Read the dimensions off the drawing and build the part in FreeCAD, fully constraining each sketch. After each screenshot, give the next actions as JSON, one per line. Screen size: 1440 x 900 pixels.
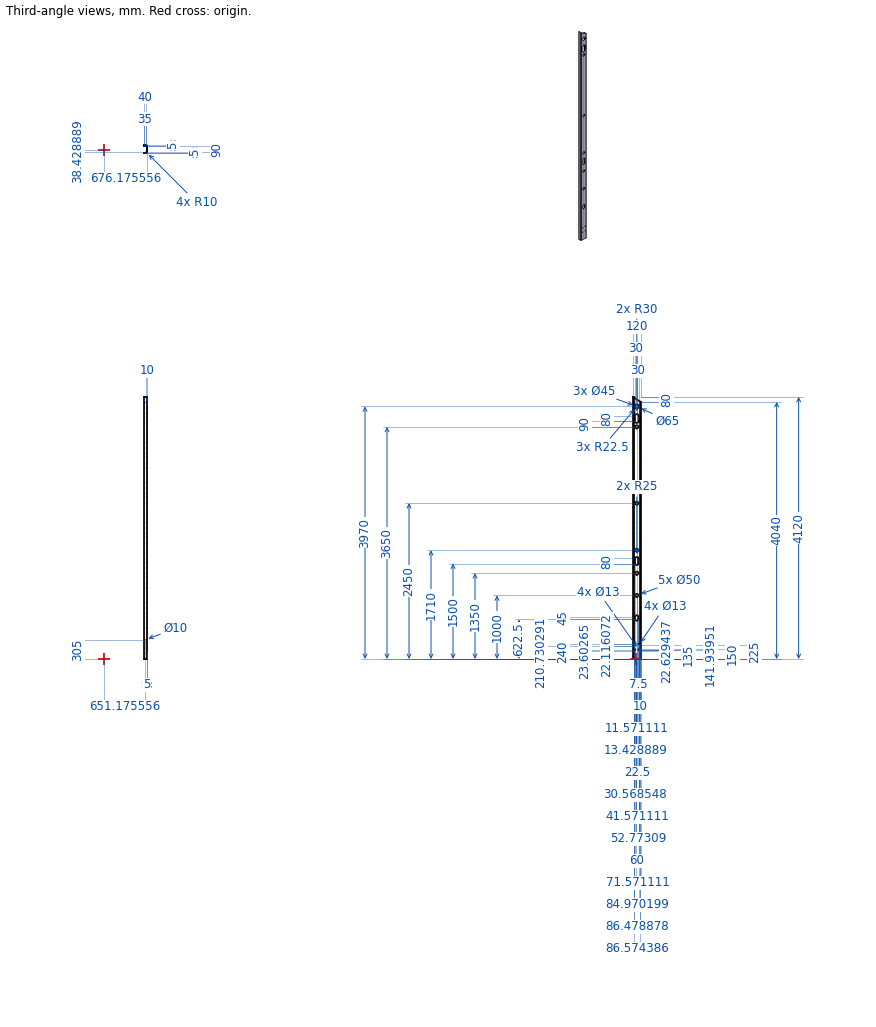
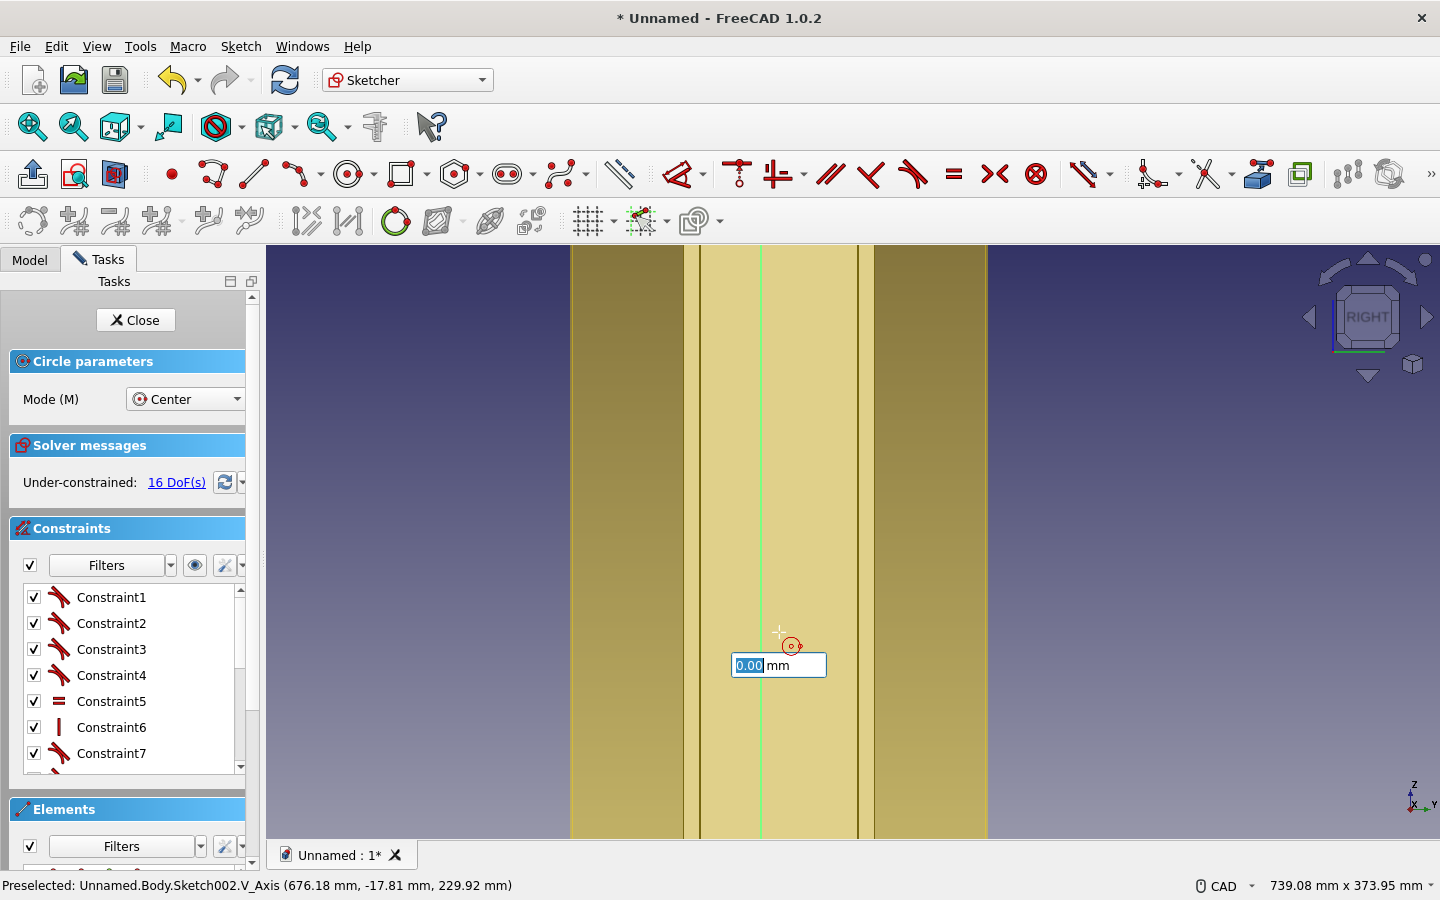
{"action": "scroll", "coordinate": [785, 639], "scroll_direction": "down", "scroll_amount": 14}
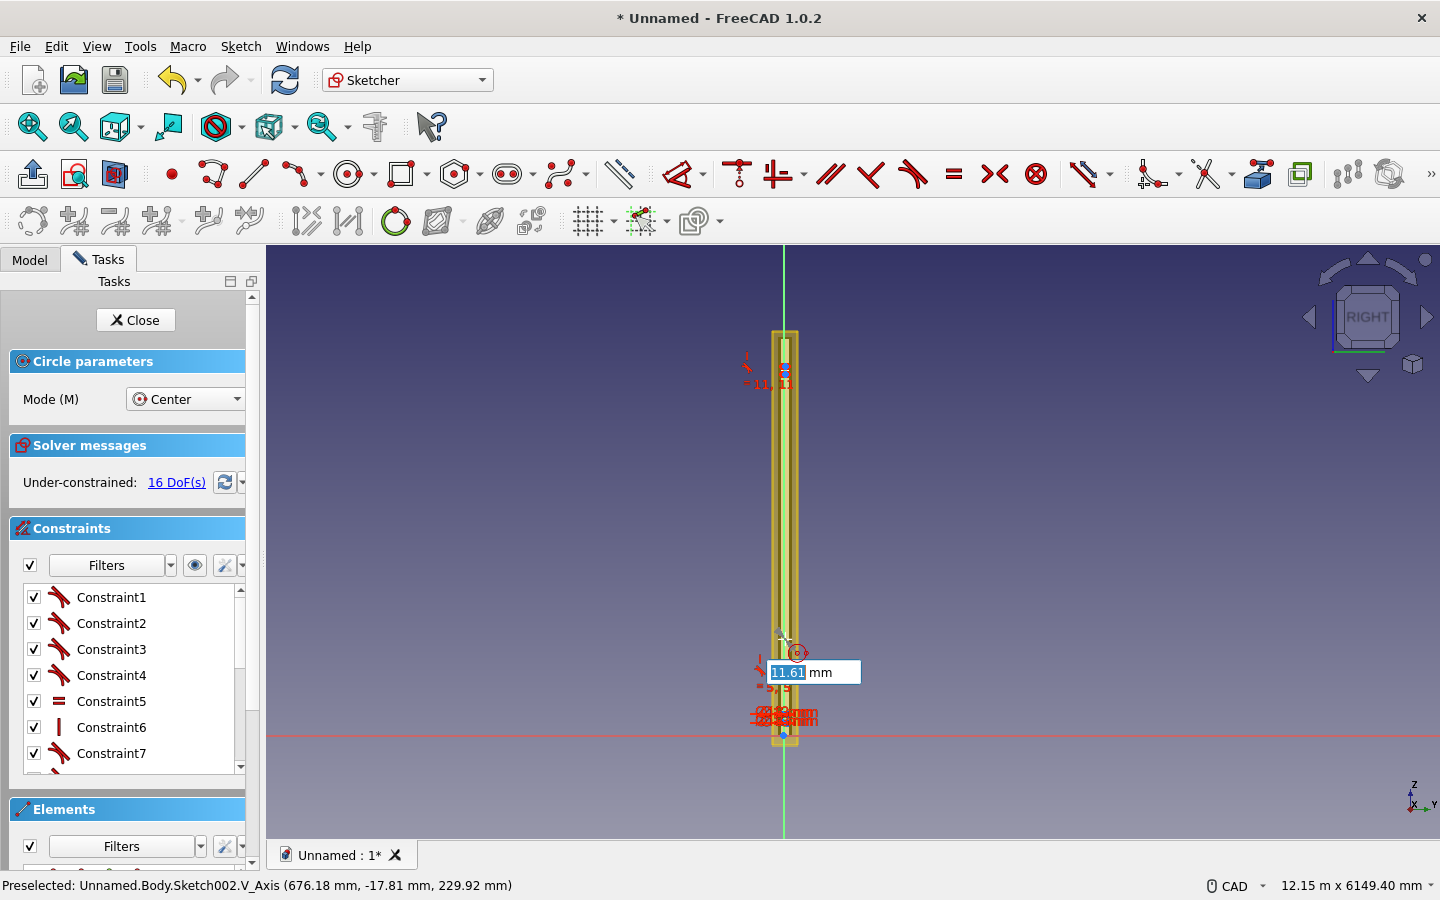
{"action": "scroll", "coordinate": [787, 638], "scroll_direction": "up", "scroll_amount": 9}
{"action": "mouse_move", "coordinate": [783, 632]}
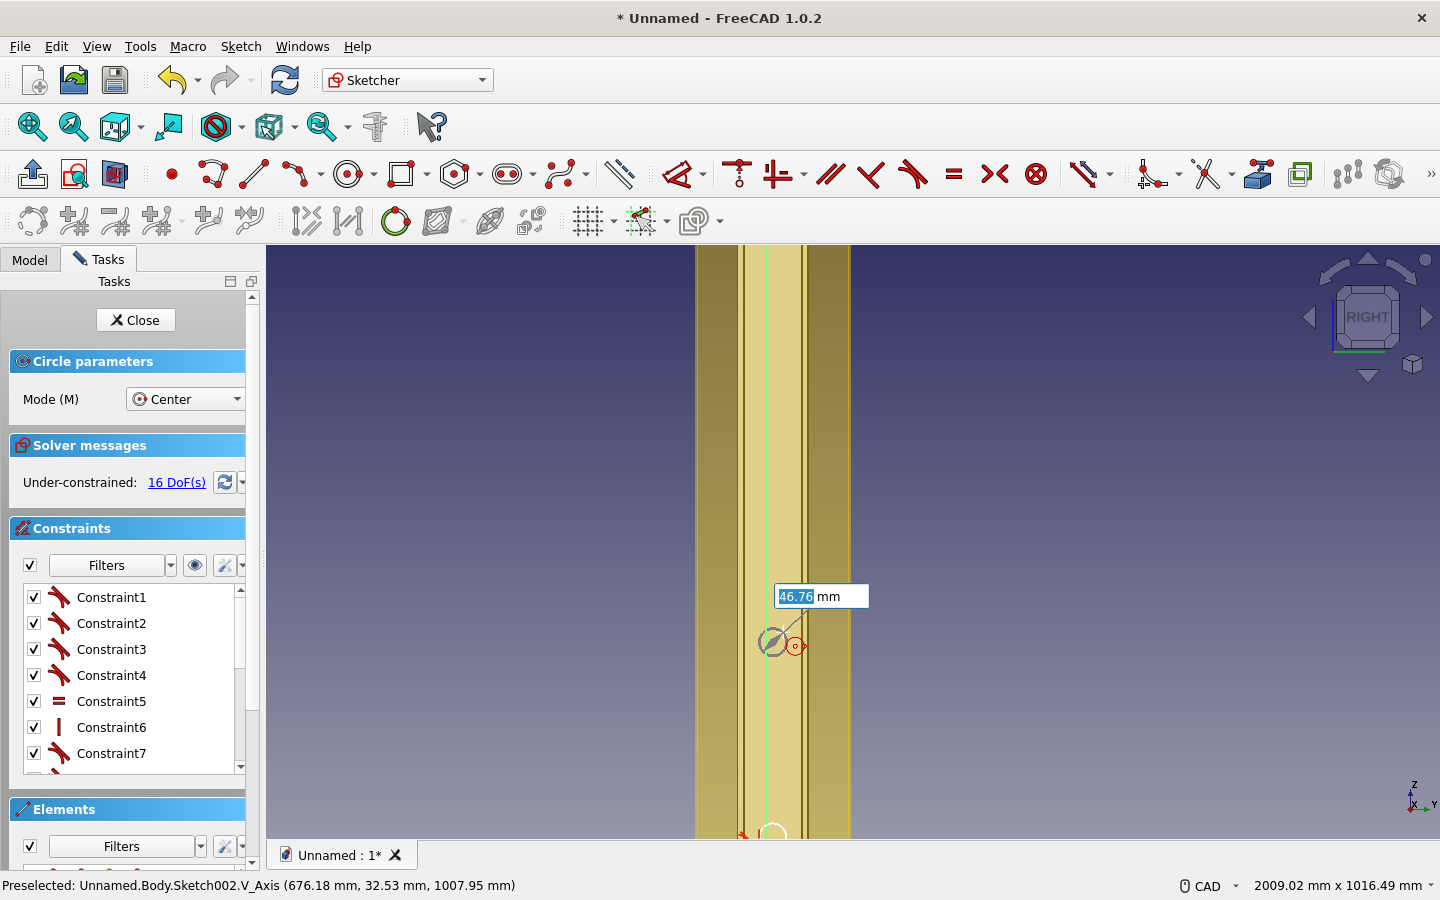
{"action": "type", "text": "50"}
{"action": "key", "text": "Return"}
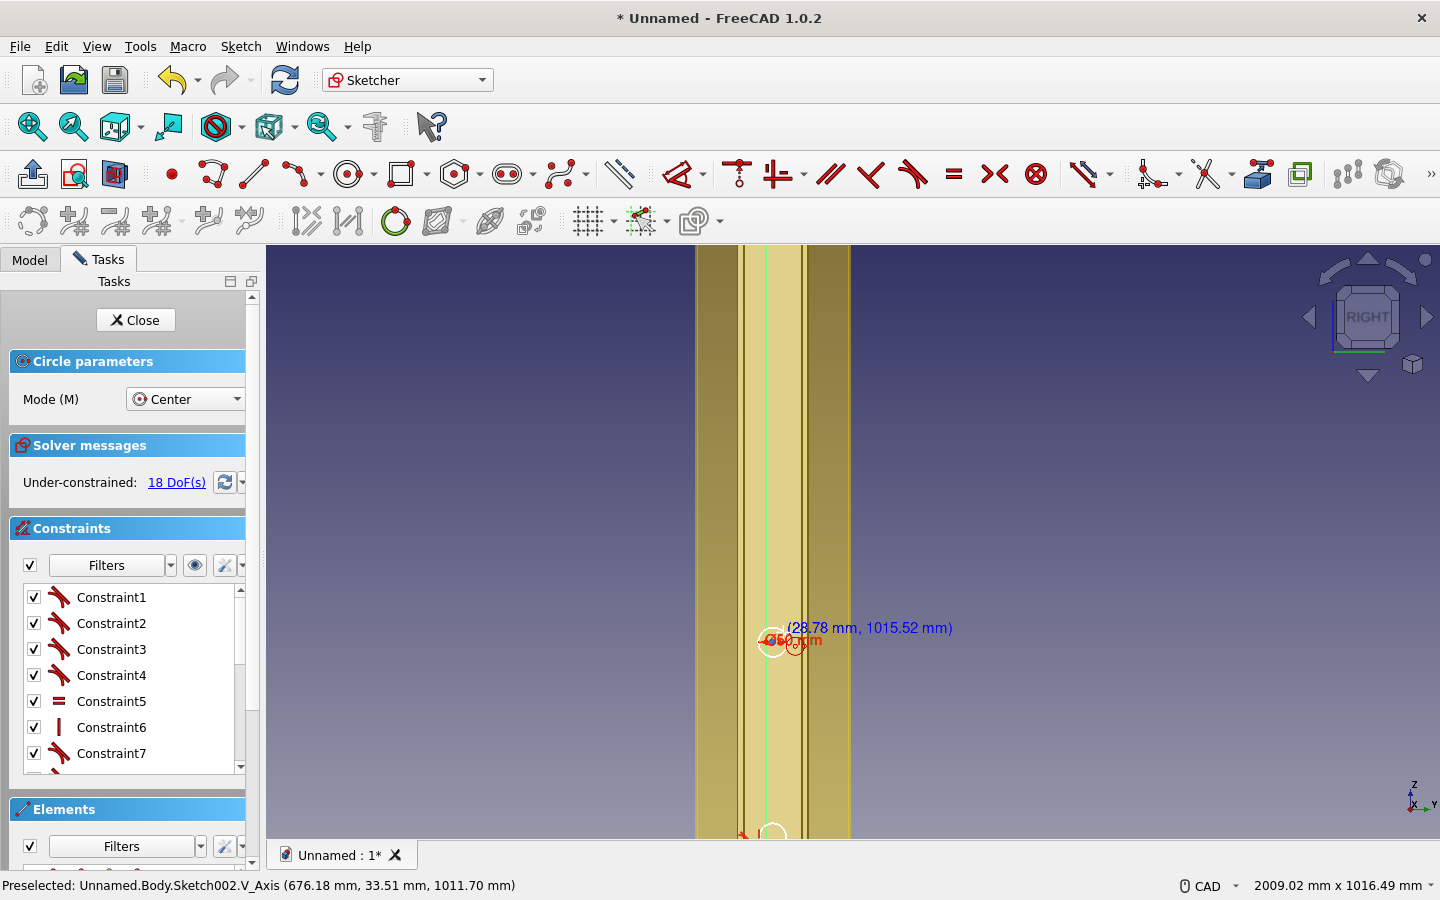
{"action": "scroll", "coordinate": [773, 438], "scroll_direction": "up", "scroll_amount": 5}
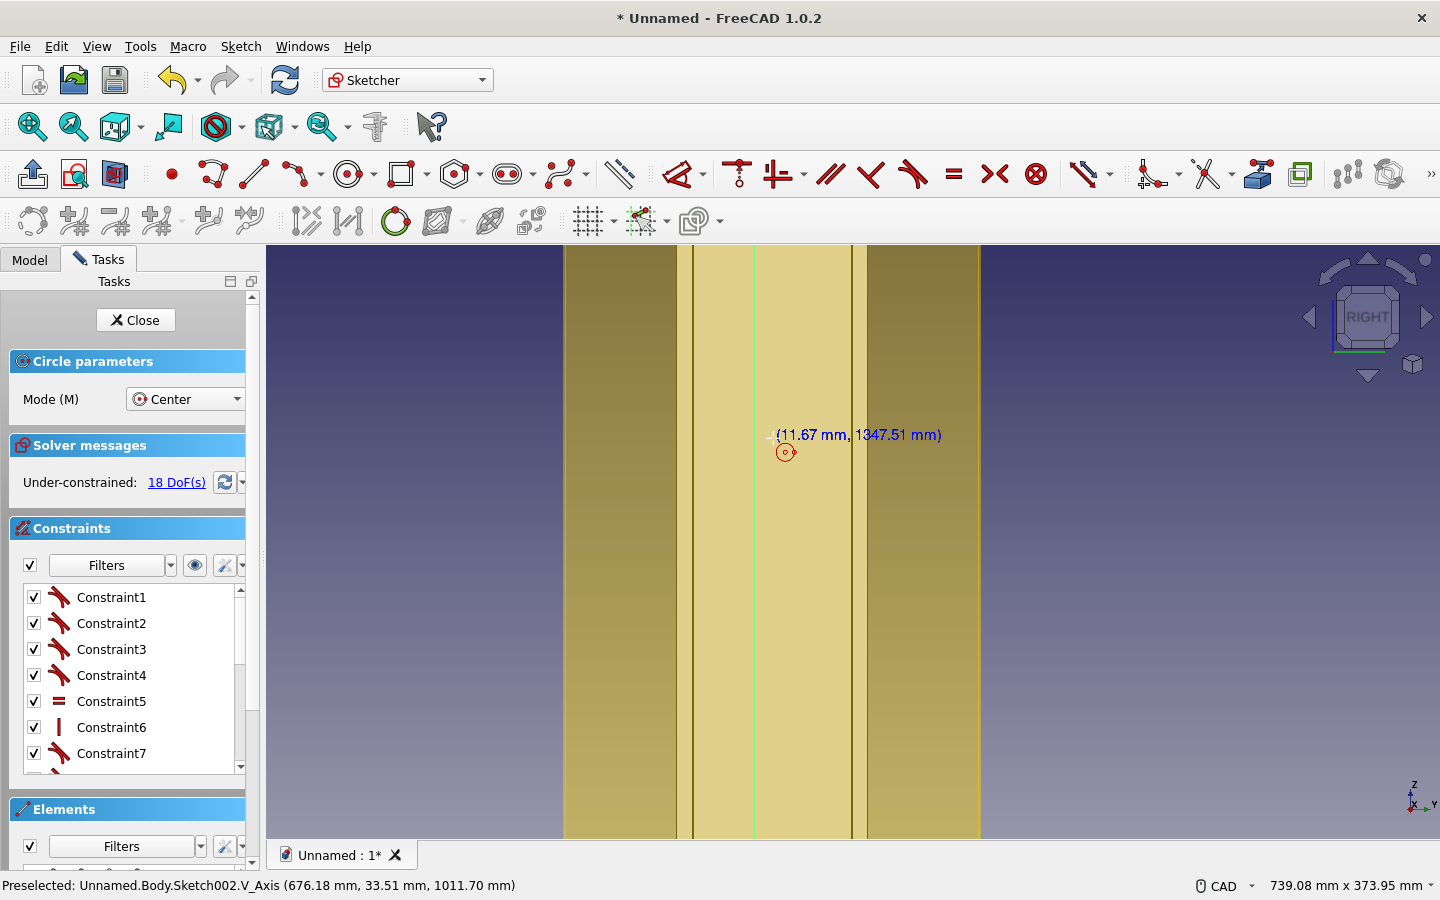
{"action": "left_click", "coordinate": [772, 436]}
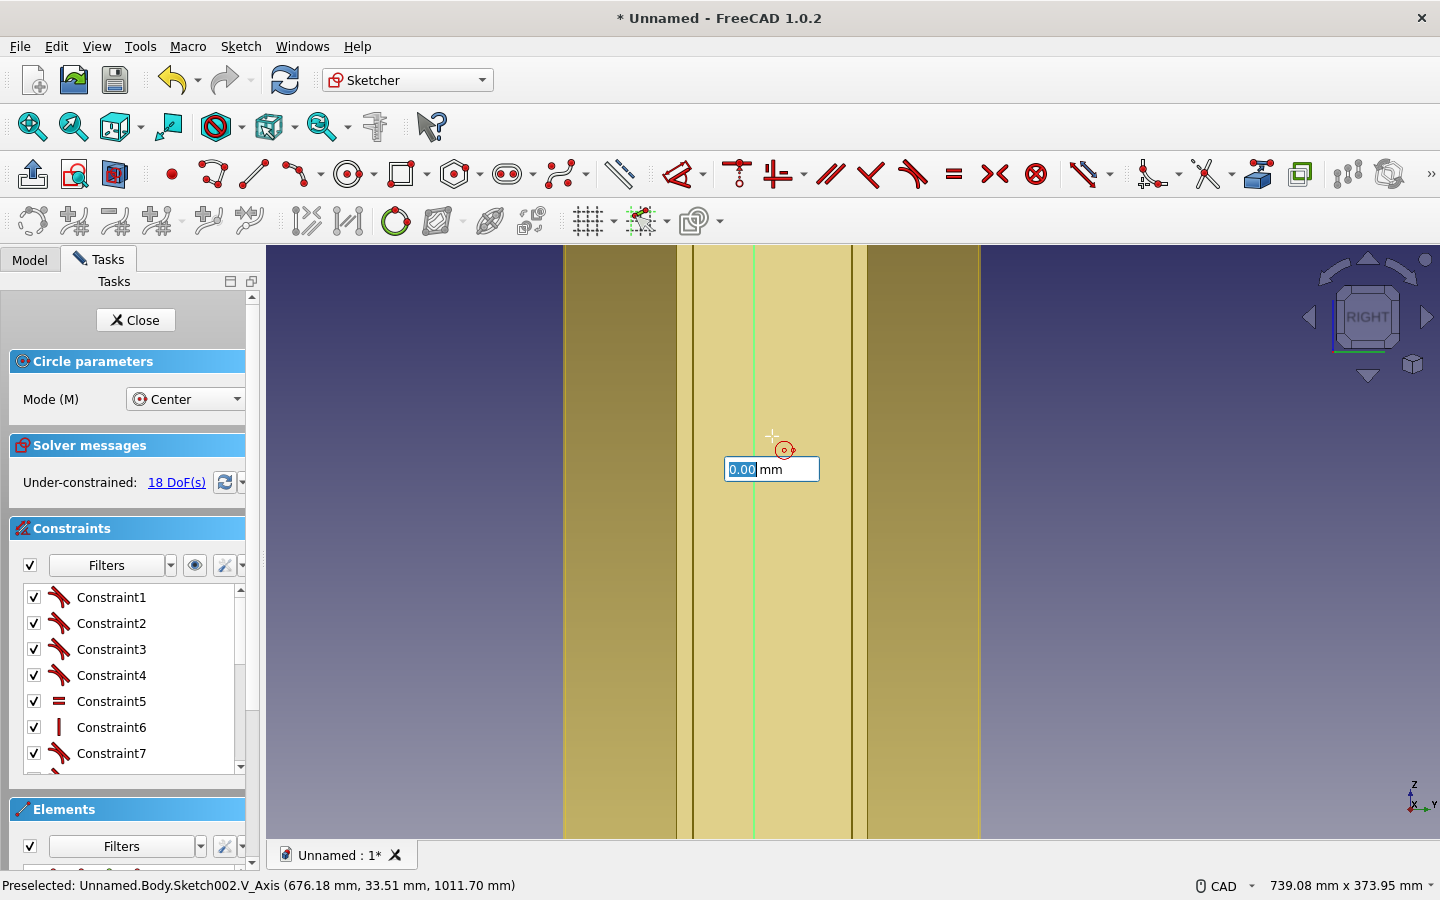
{"action": "scroll", "coordinate": [785, 615], "scroll_direction": "down", "scroll_amount": 14}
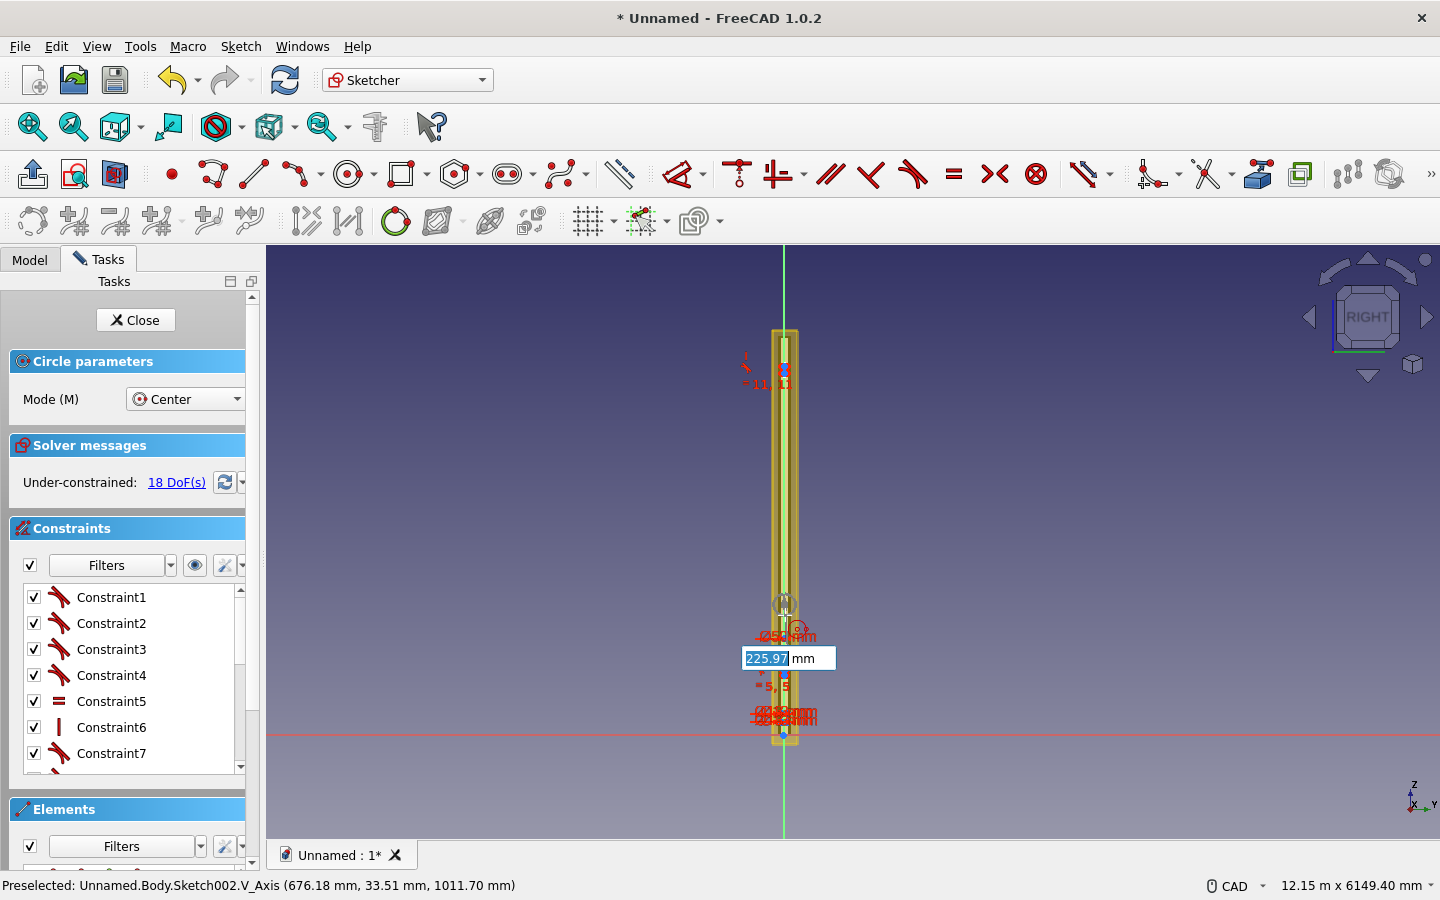
{"action": "scroll", "coordinate": [786, 603], "scroll_direction": "up", "scroll_amount": 9}
{"action": "mouse_move", "coordinate": [786, 600]}